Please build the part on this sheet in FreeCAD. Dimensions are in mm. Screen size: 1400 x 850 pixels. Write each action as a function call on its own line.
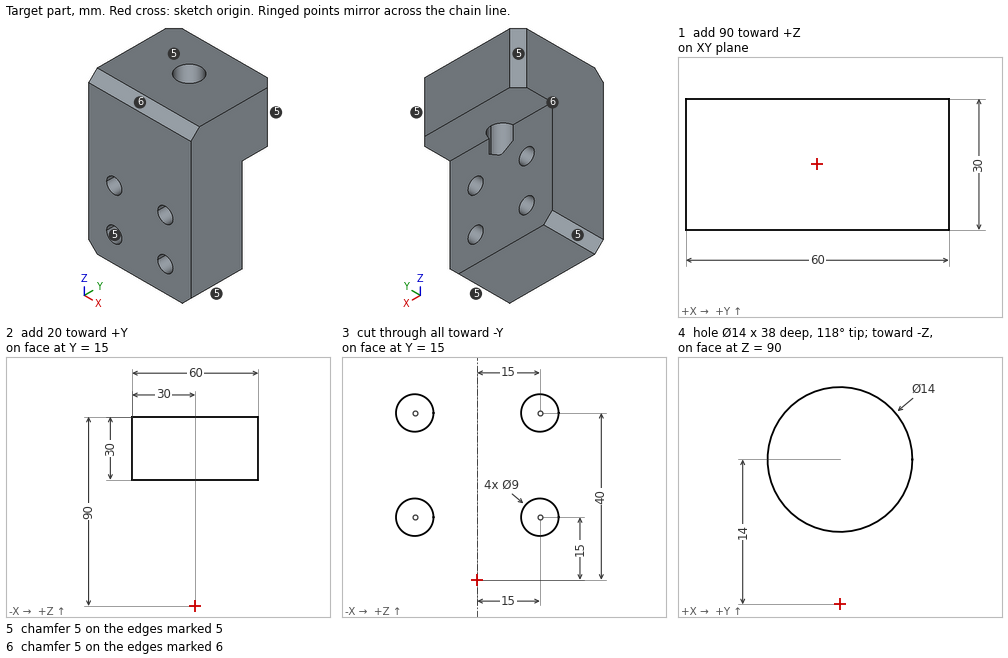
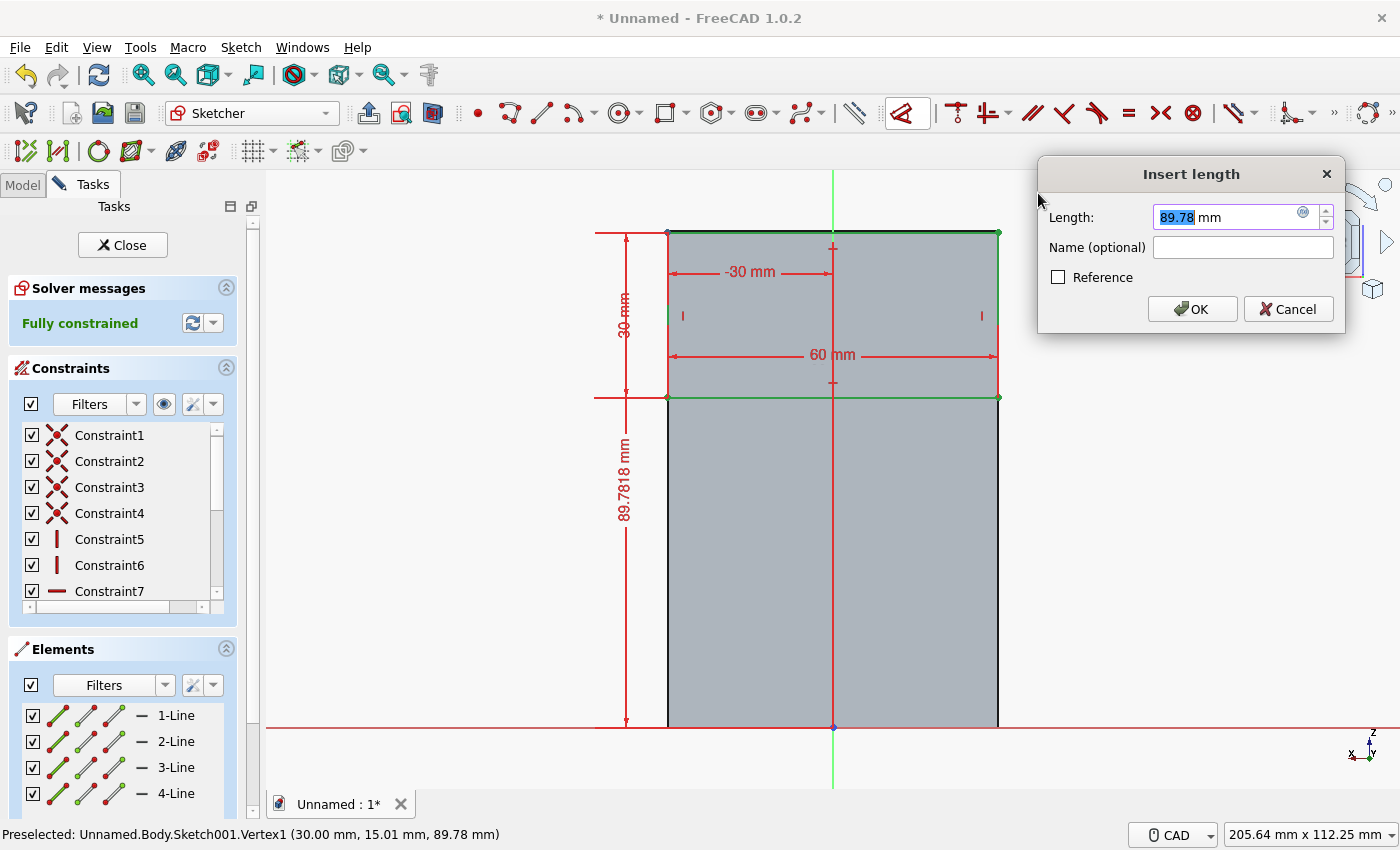
text(90)
key(Return)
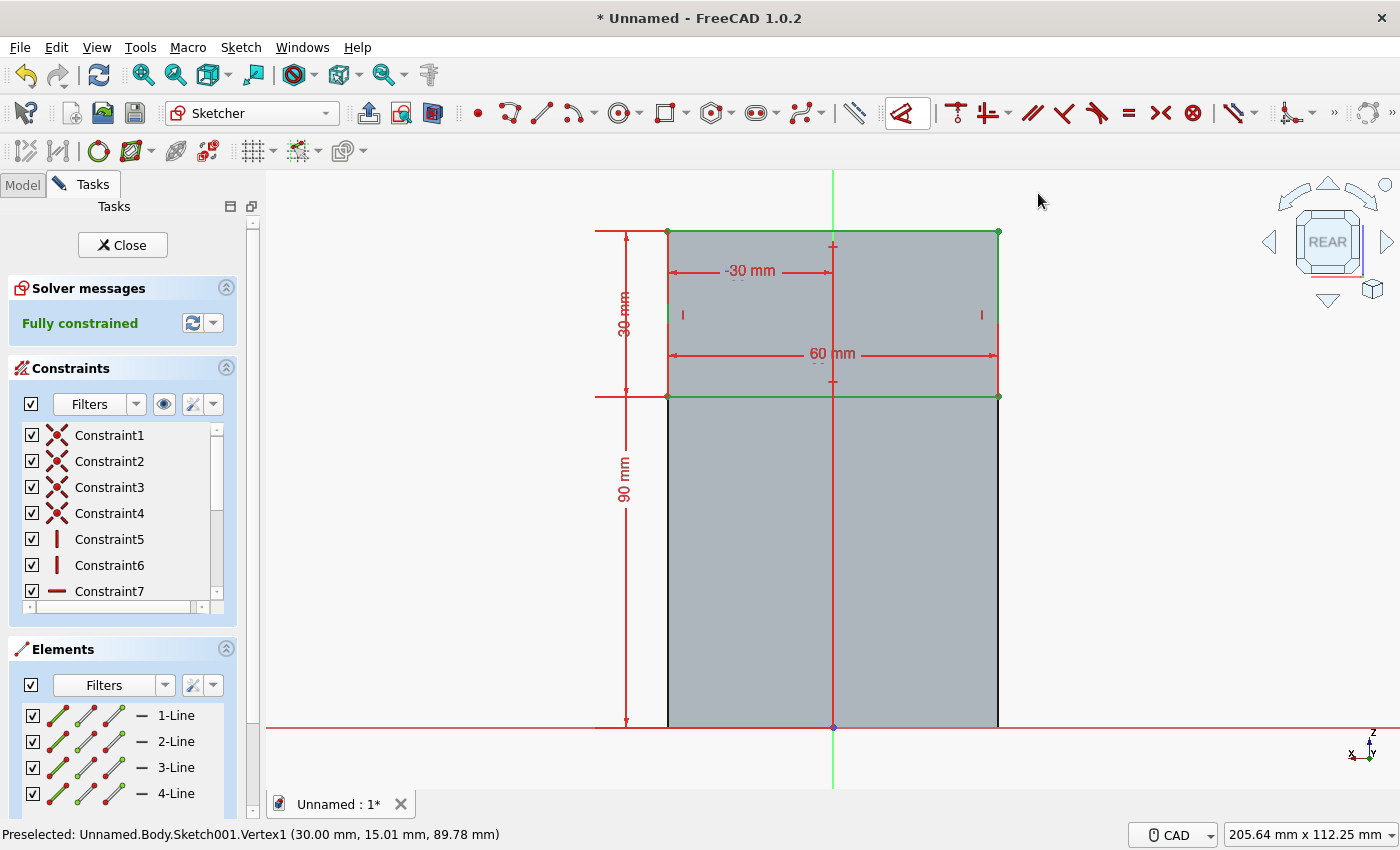
click(123, 245)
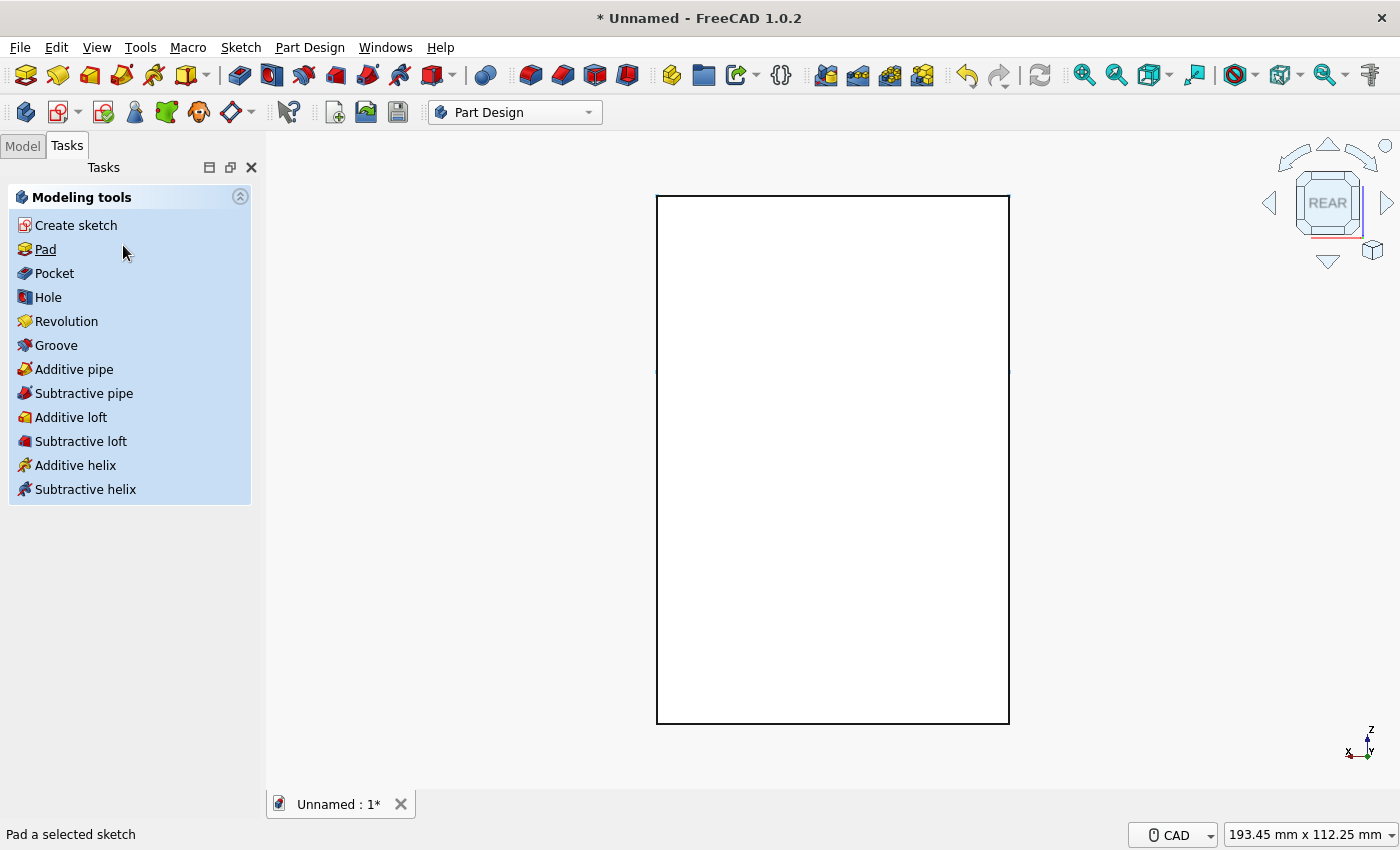
click(26, 76)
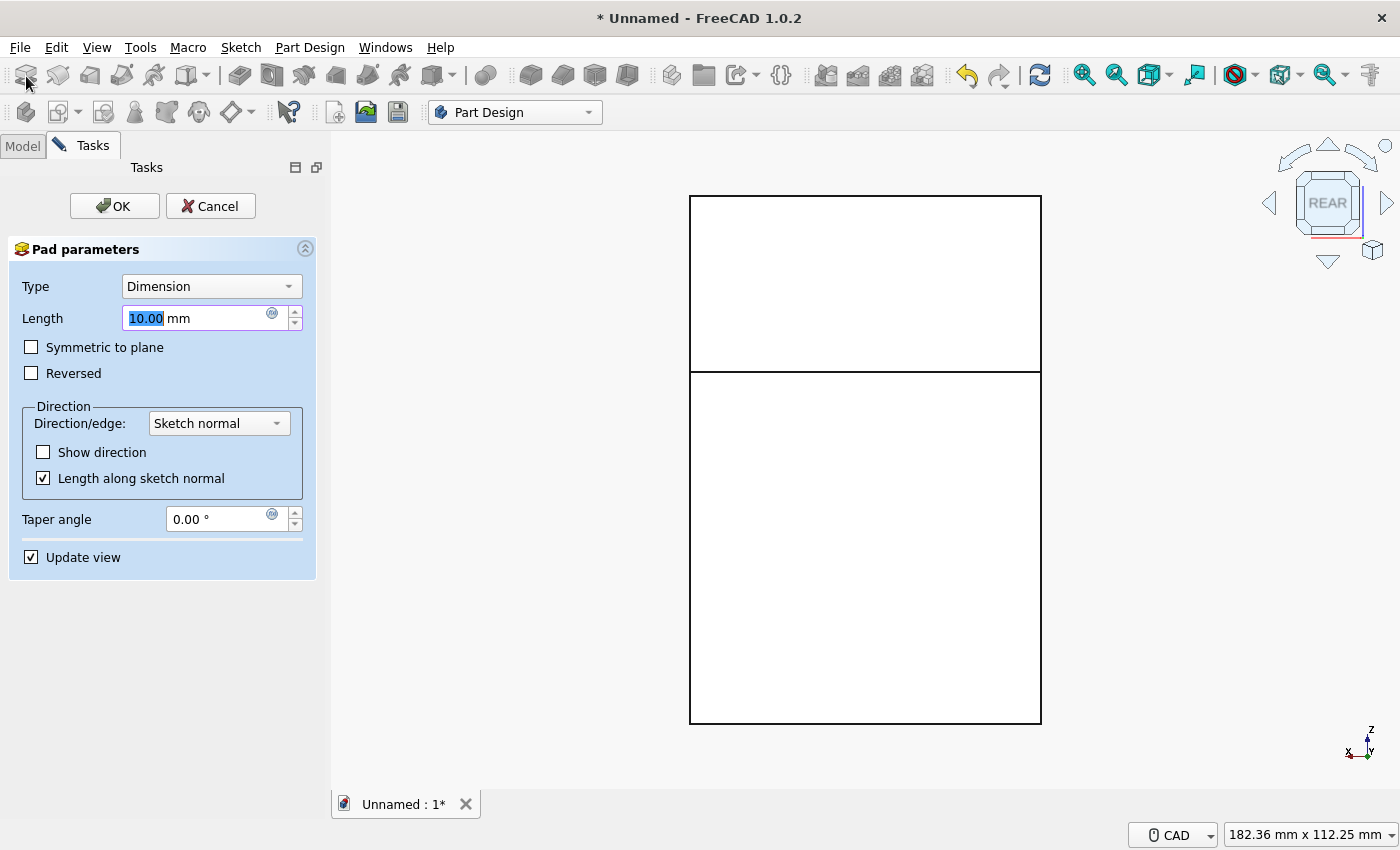
text(20)
key(Tab)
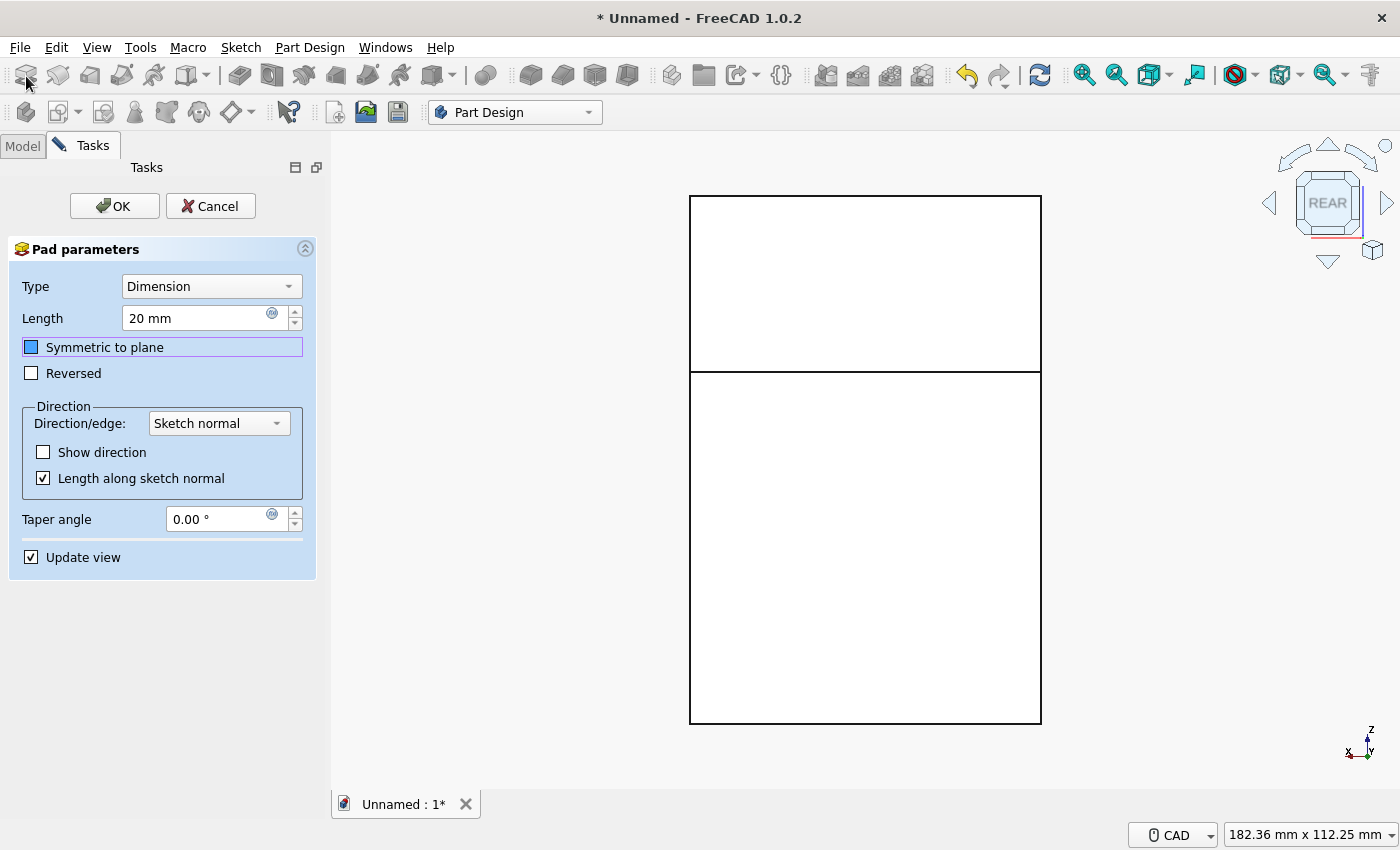
click(115, 206)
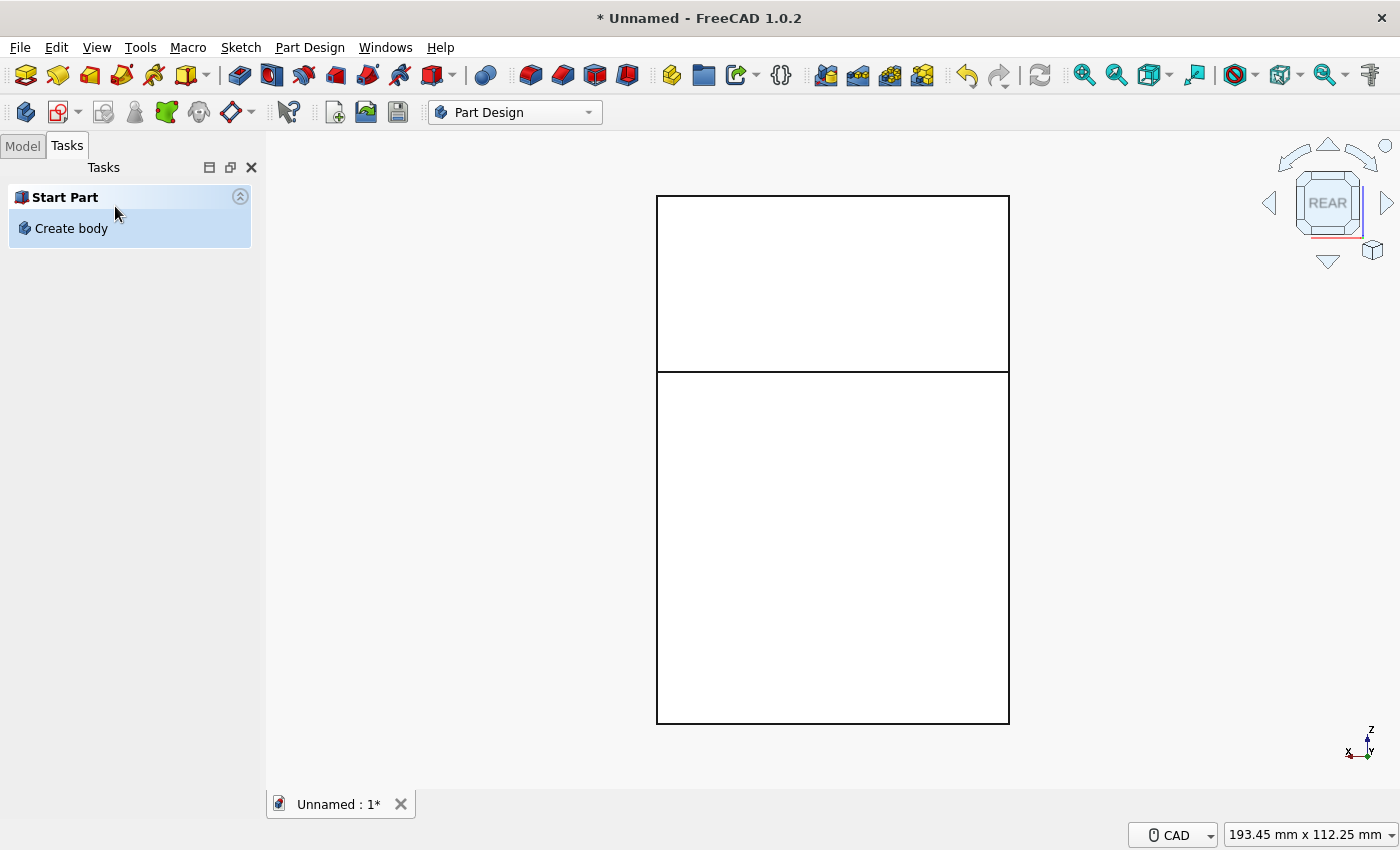
click(833, 547)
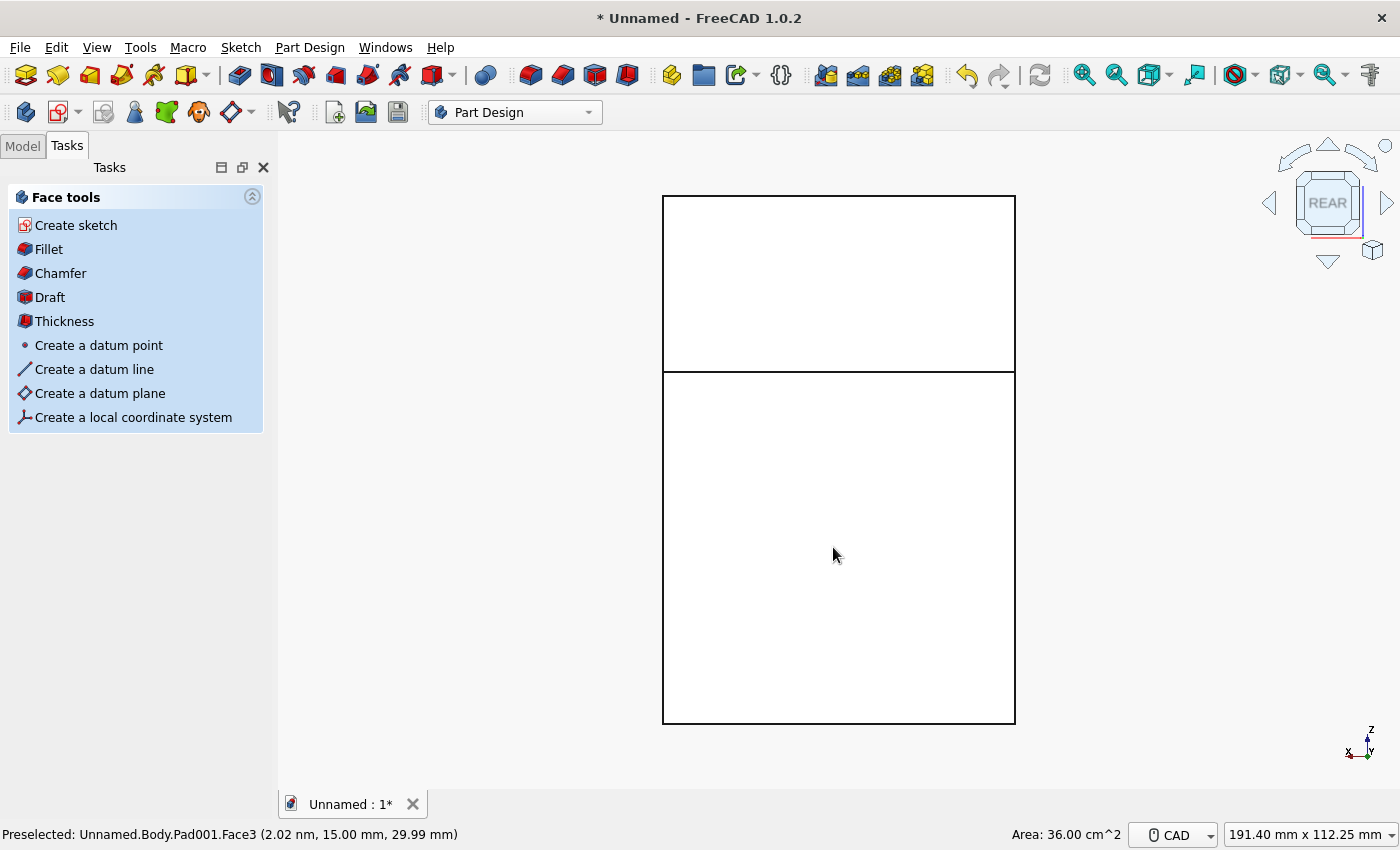
click(58, 112)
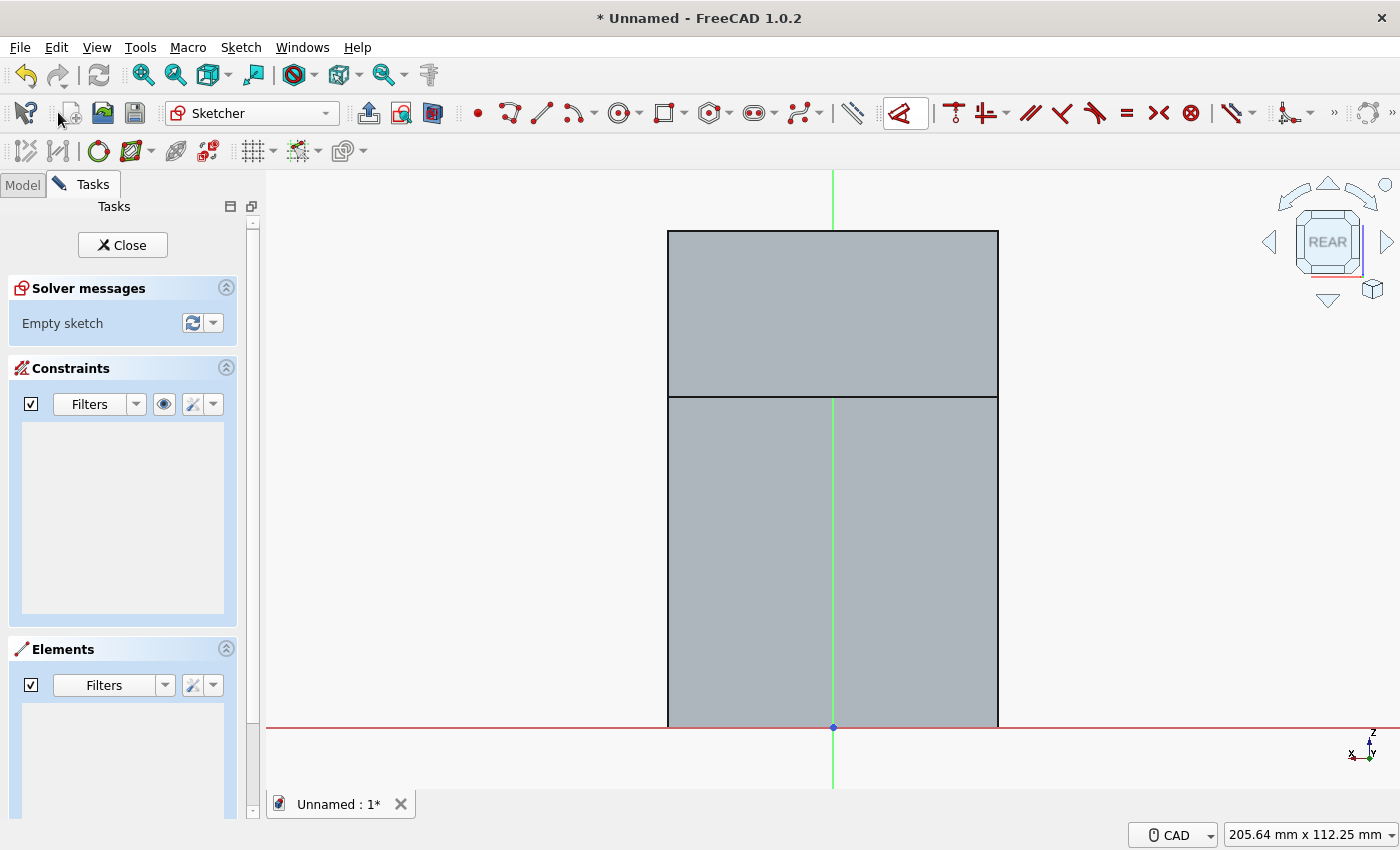
scroll(972, 761, up, 2)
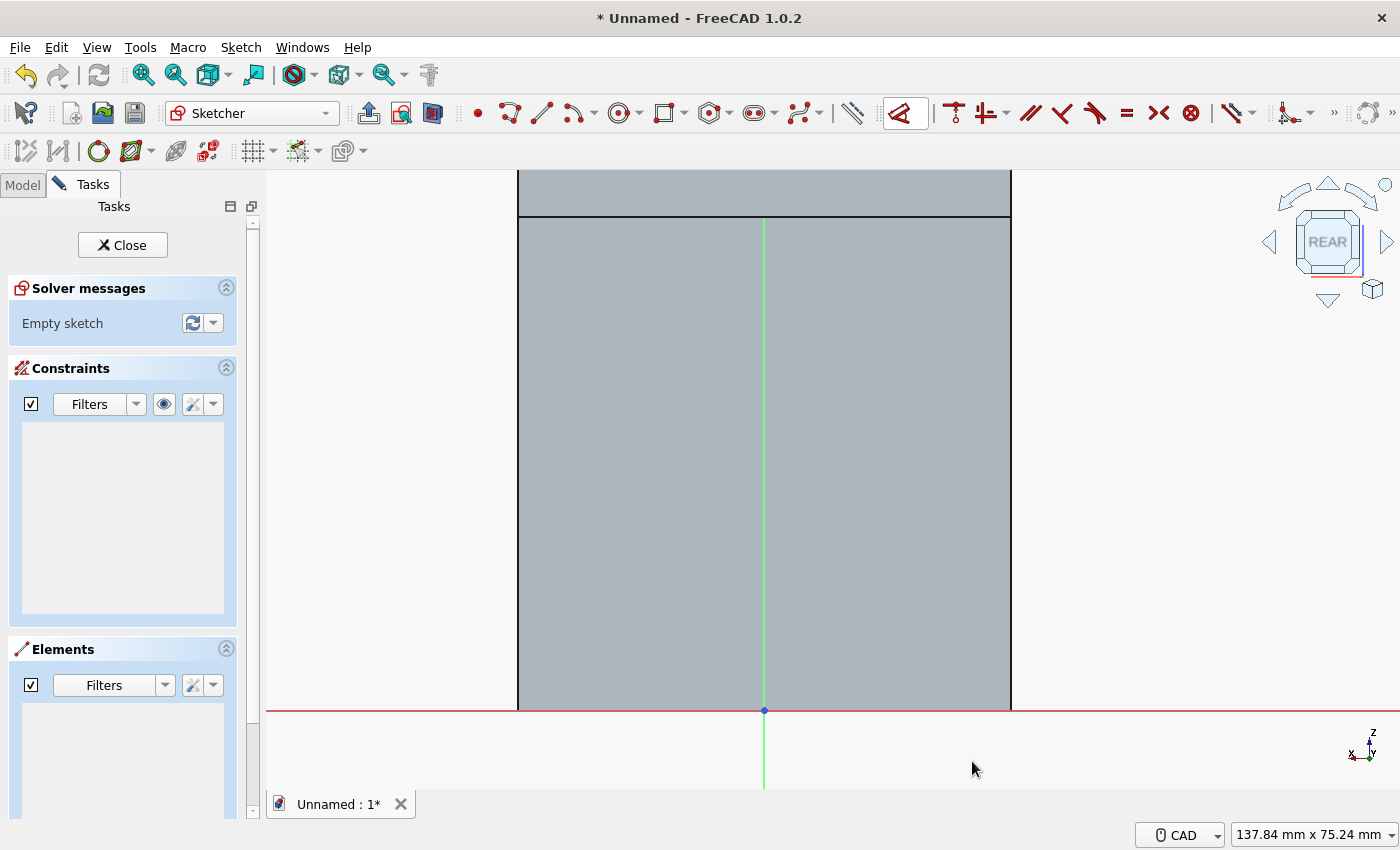
click(620, 114)